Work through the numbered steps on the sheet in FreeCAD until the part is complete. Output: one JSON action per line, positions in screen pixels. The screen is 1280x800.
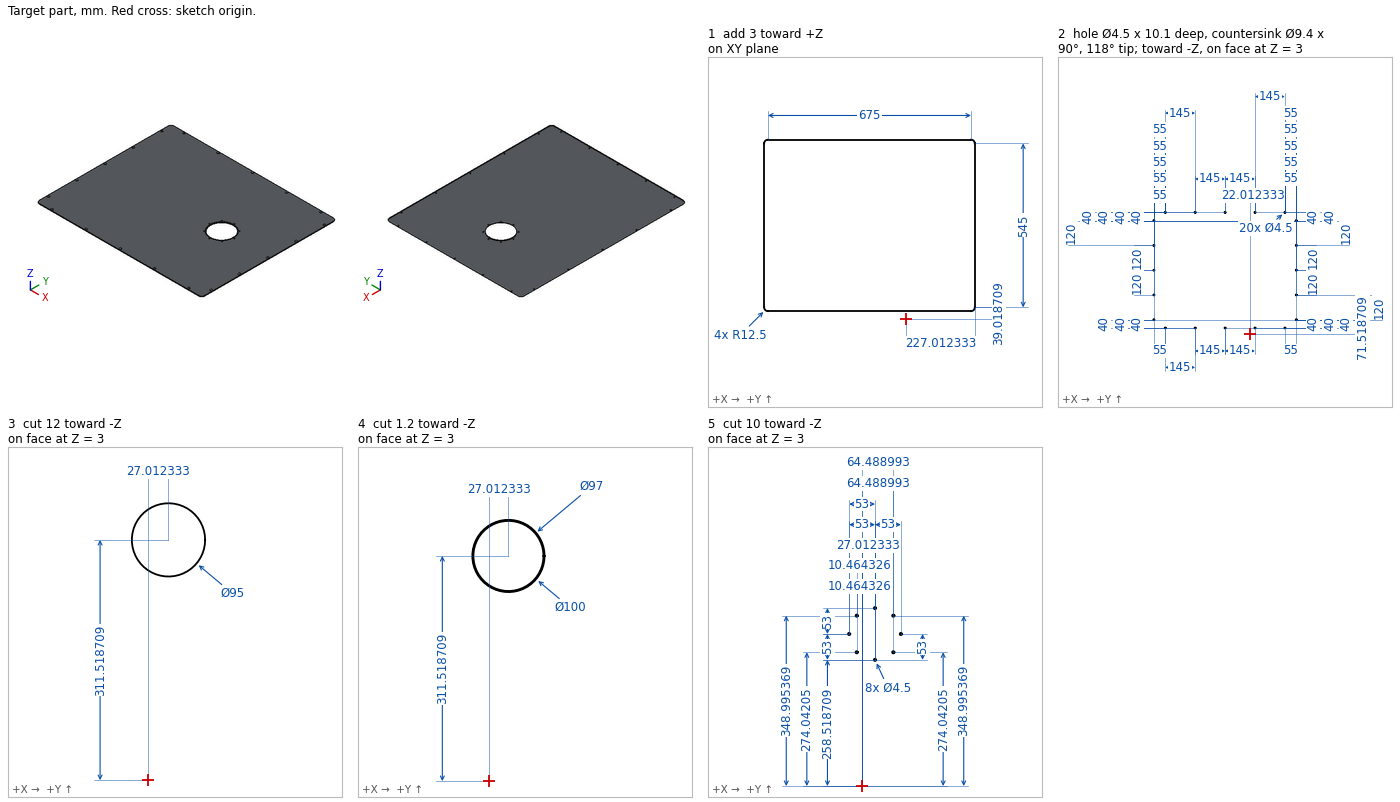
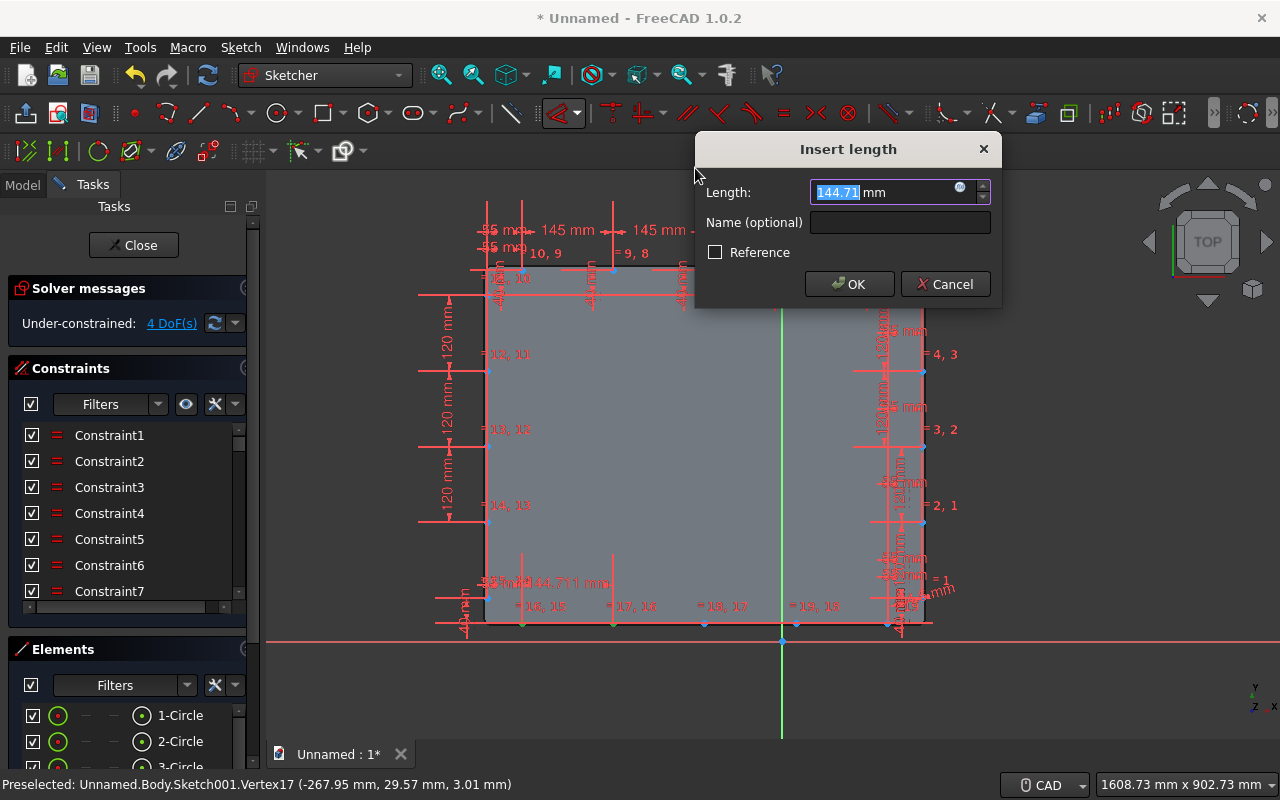
{"action": "type", "text": "145"}
{"action": "key", "text": "Return"}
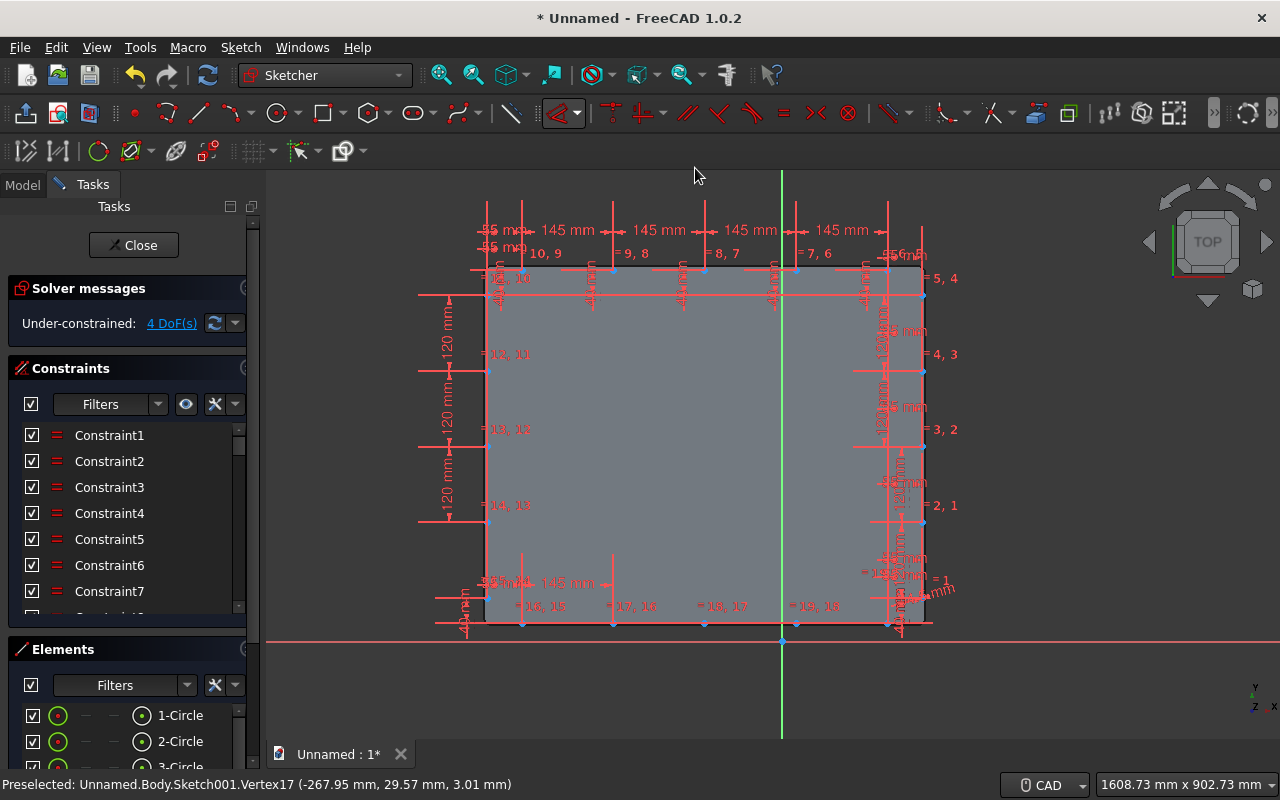
{"action": "left_click", "coordinate": [613, 623]}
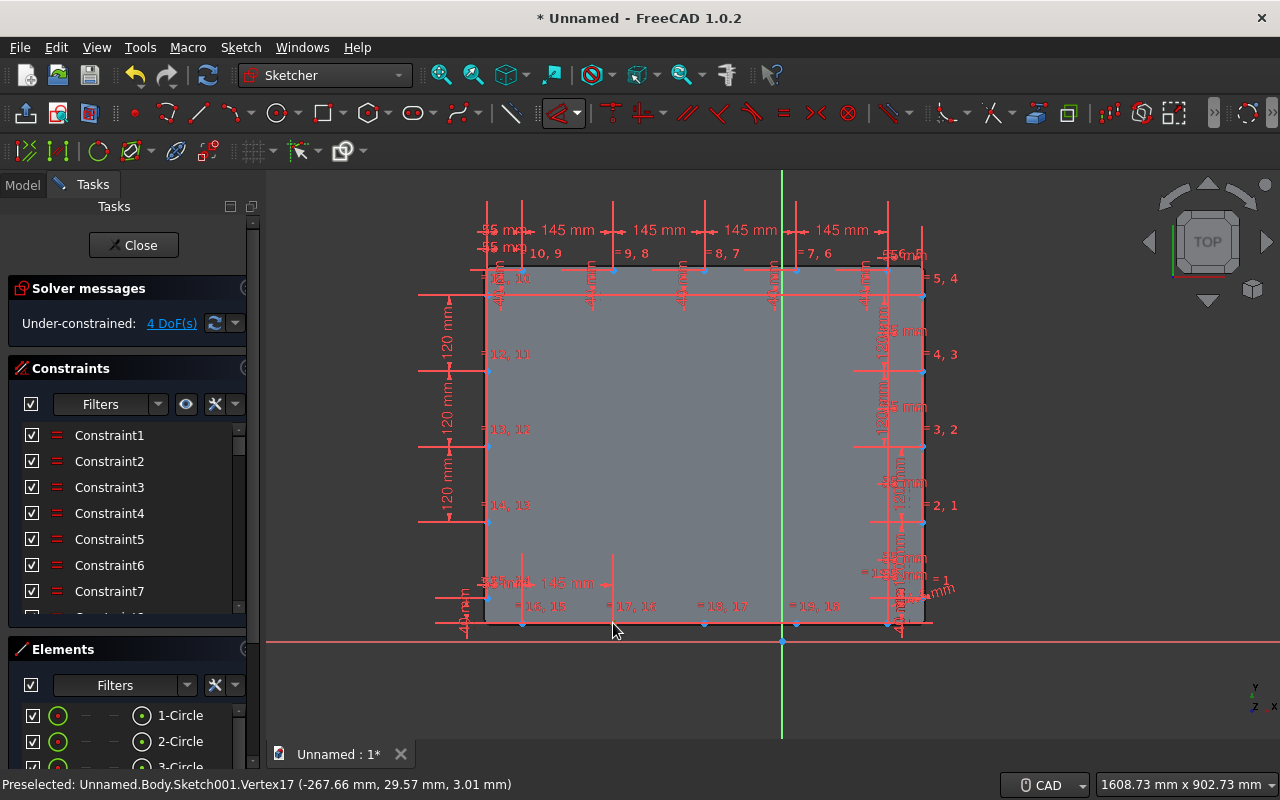
{"action": "left_click", "coordinate": [704, 623]}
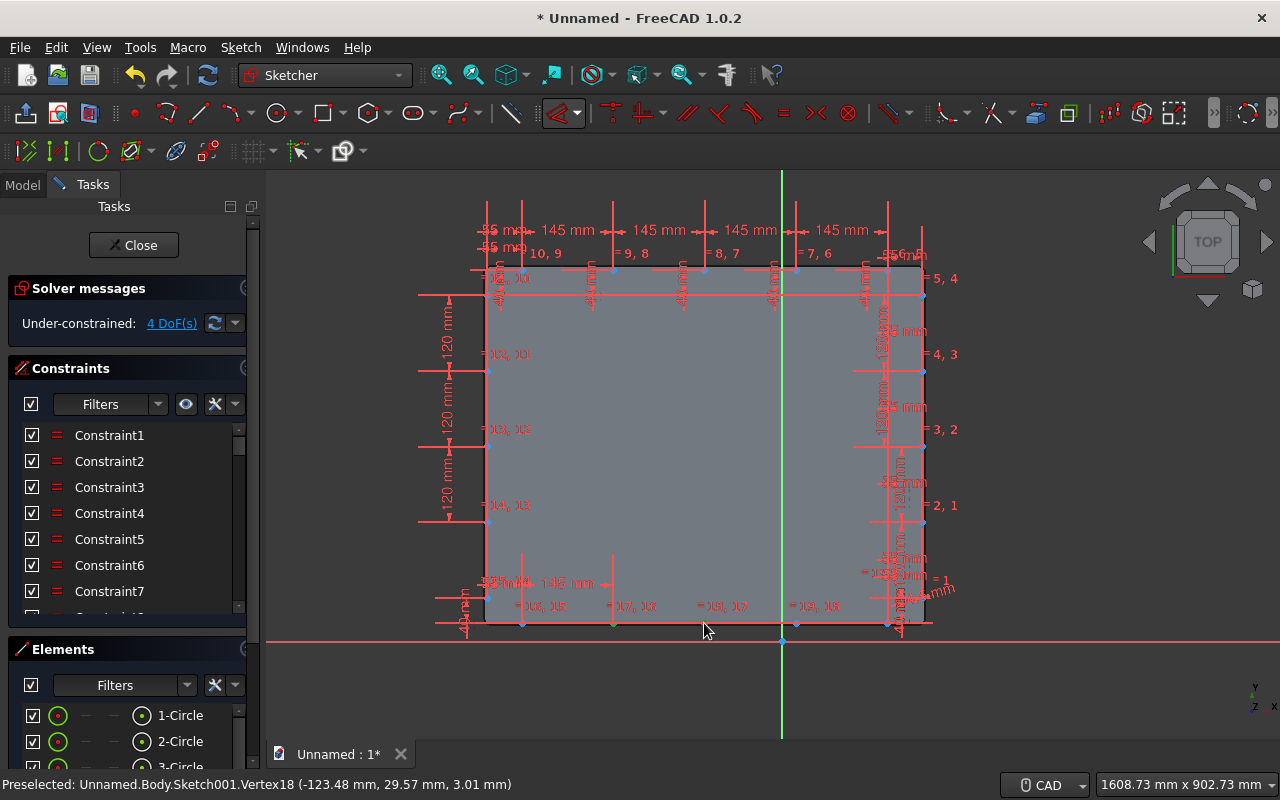
{"action": "left_click", "coordinate": [580, 114]}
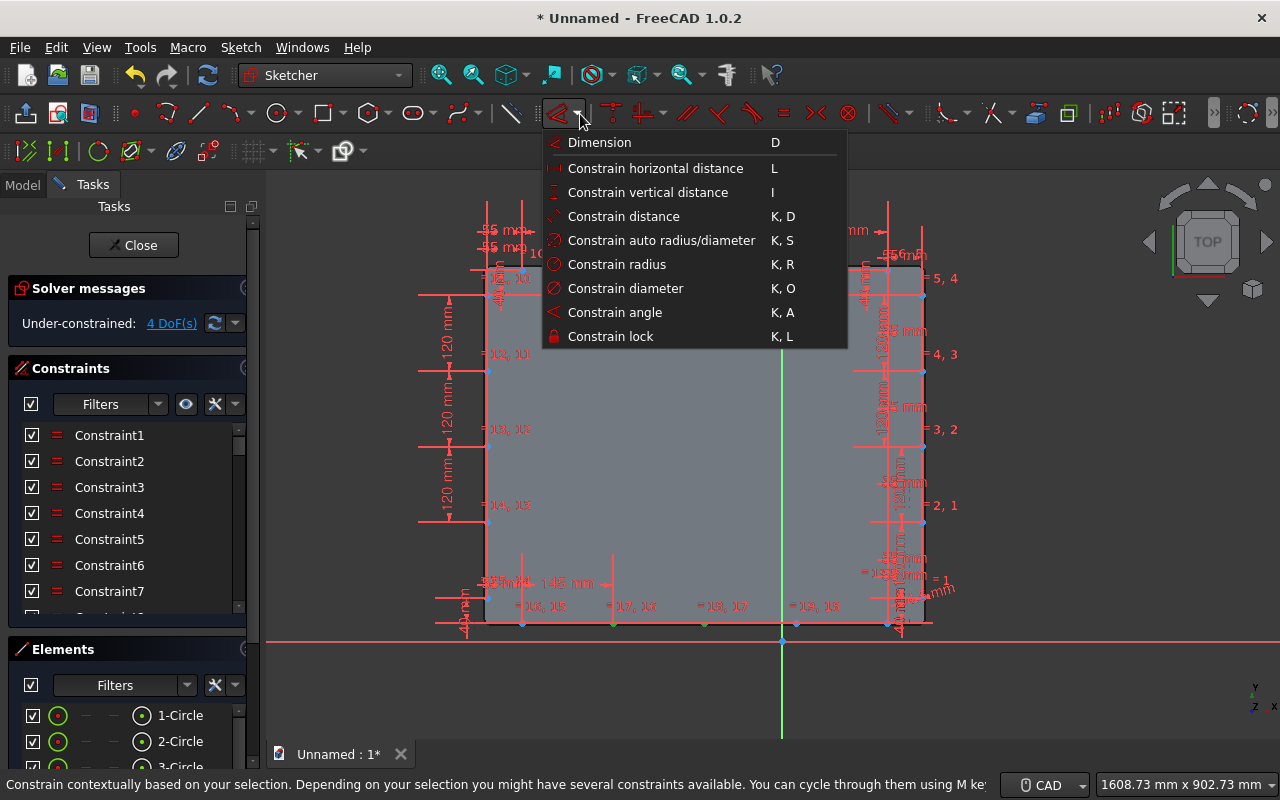
{"action": "left_click", "coordinate": [695, 168]}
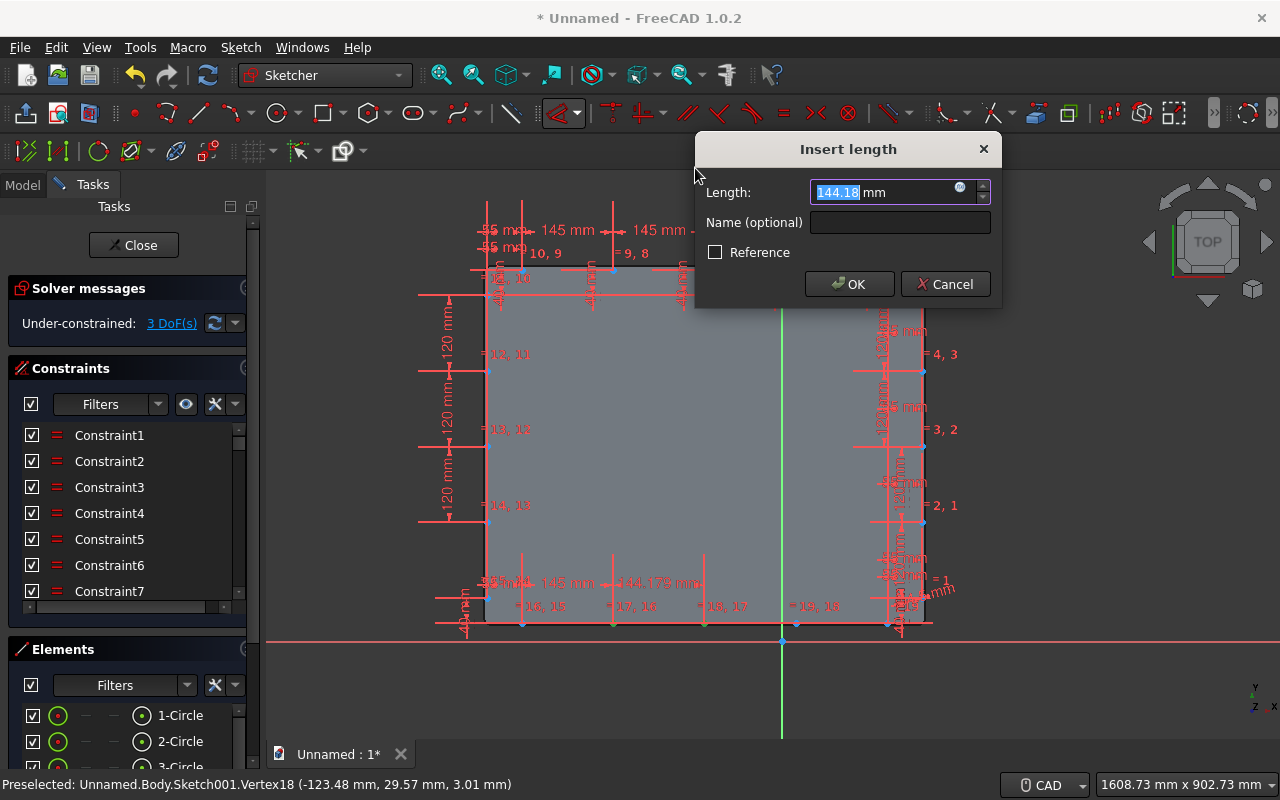
{"action": "type", "text": "145"}
{"action": "key", "text": "Return"}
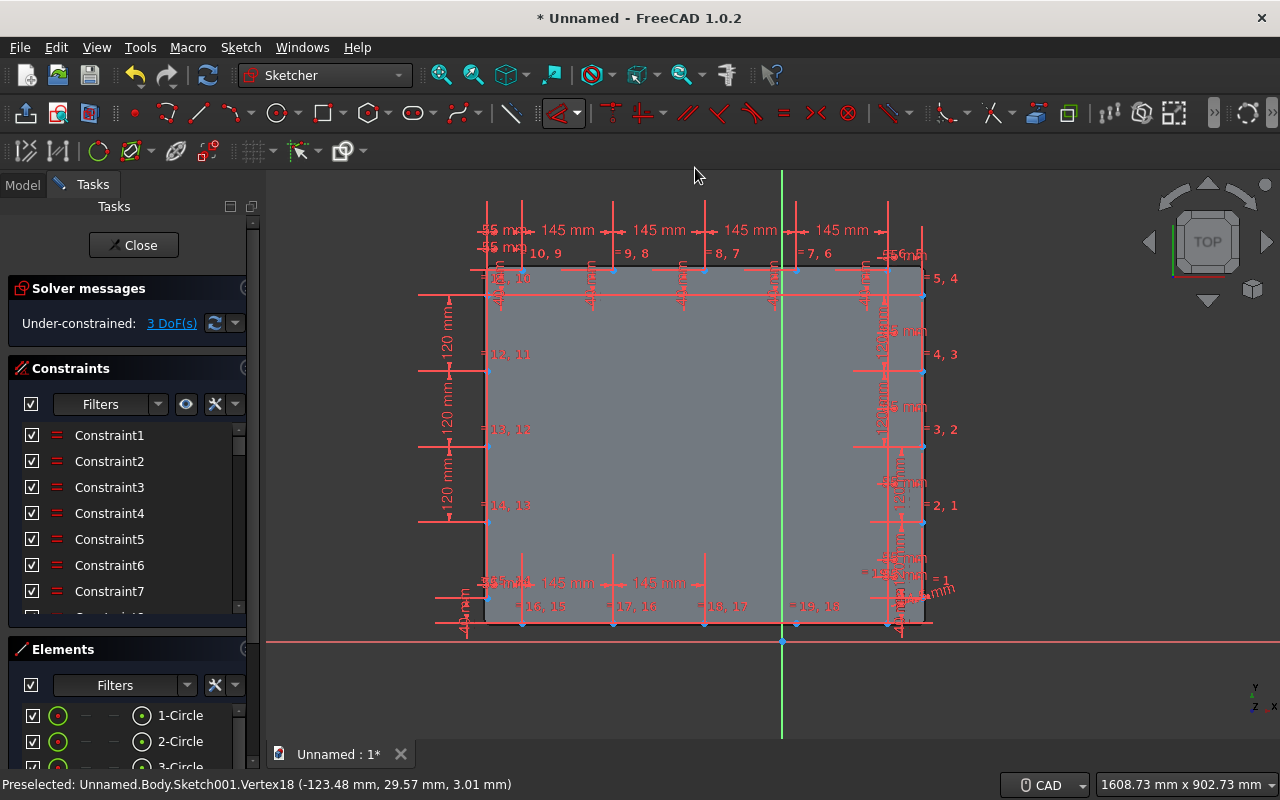
{"action": "left_click", "coordinate": [705, 623]}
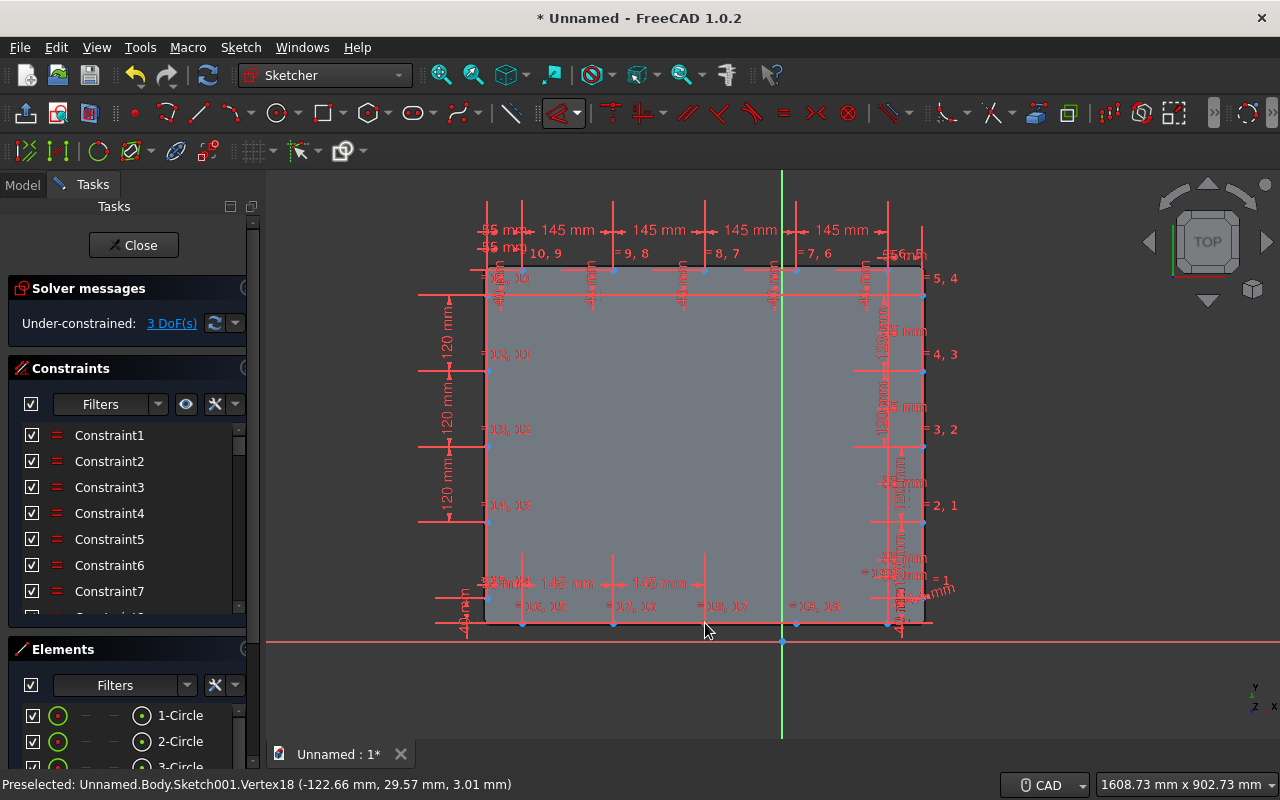
{"action": "left_click", "coordinate": [796, 623]}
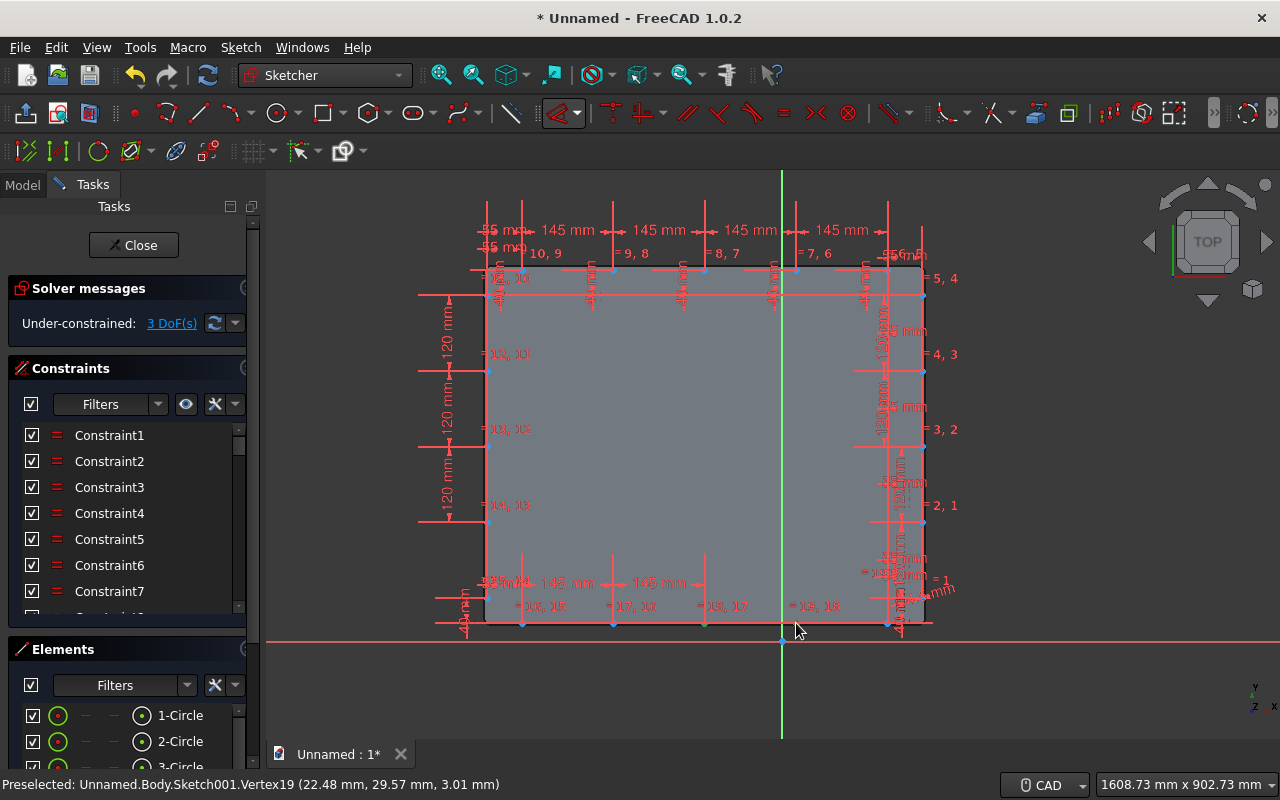
{"action": "left_click", "coordinate": [580, 114]}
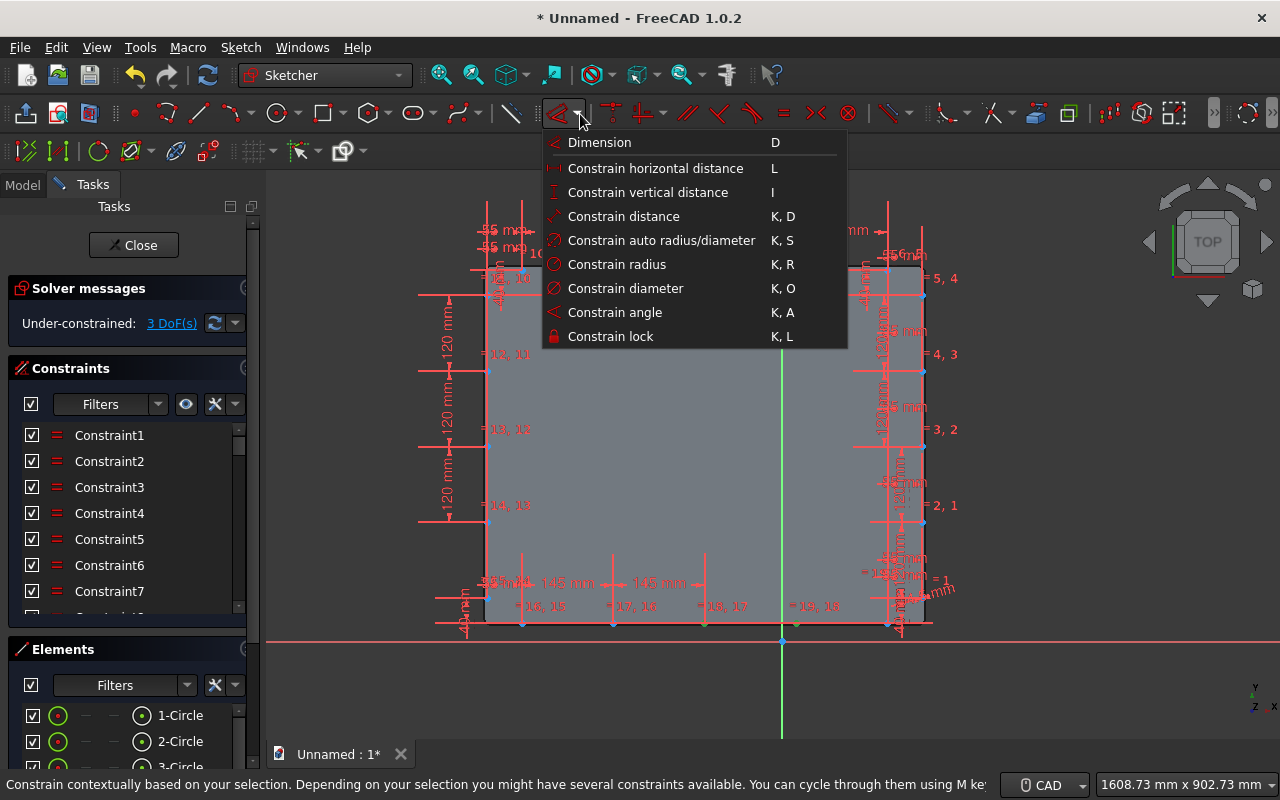
{"action": "left_click", "coordinate": [695, 168]}